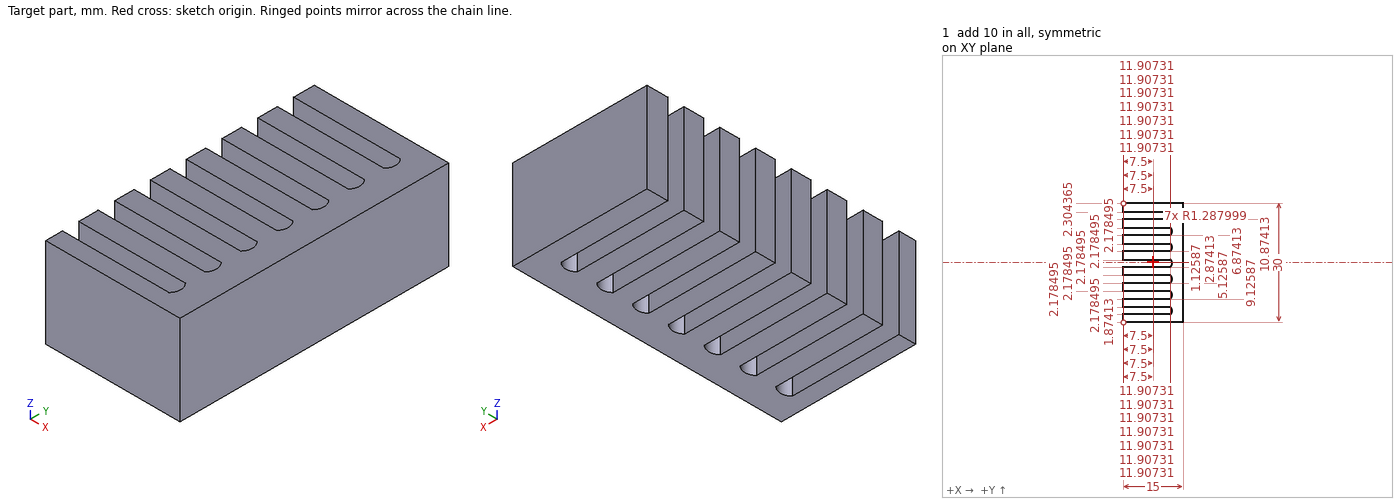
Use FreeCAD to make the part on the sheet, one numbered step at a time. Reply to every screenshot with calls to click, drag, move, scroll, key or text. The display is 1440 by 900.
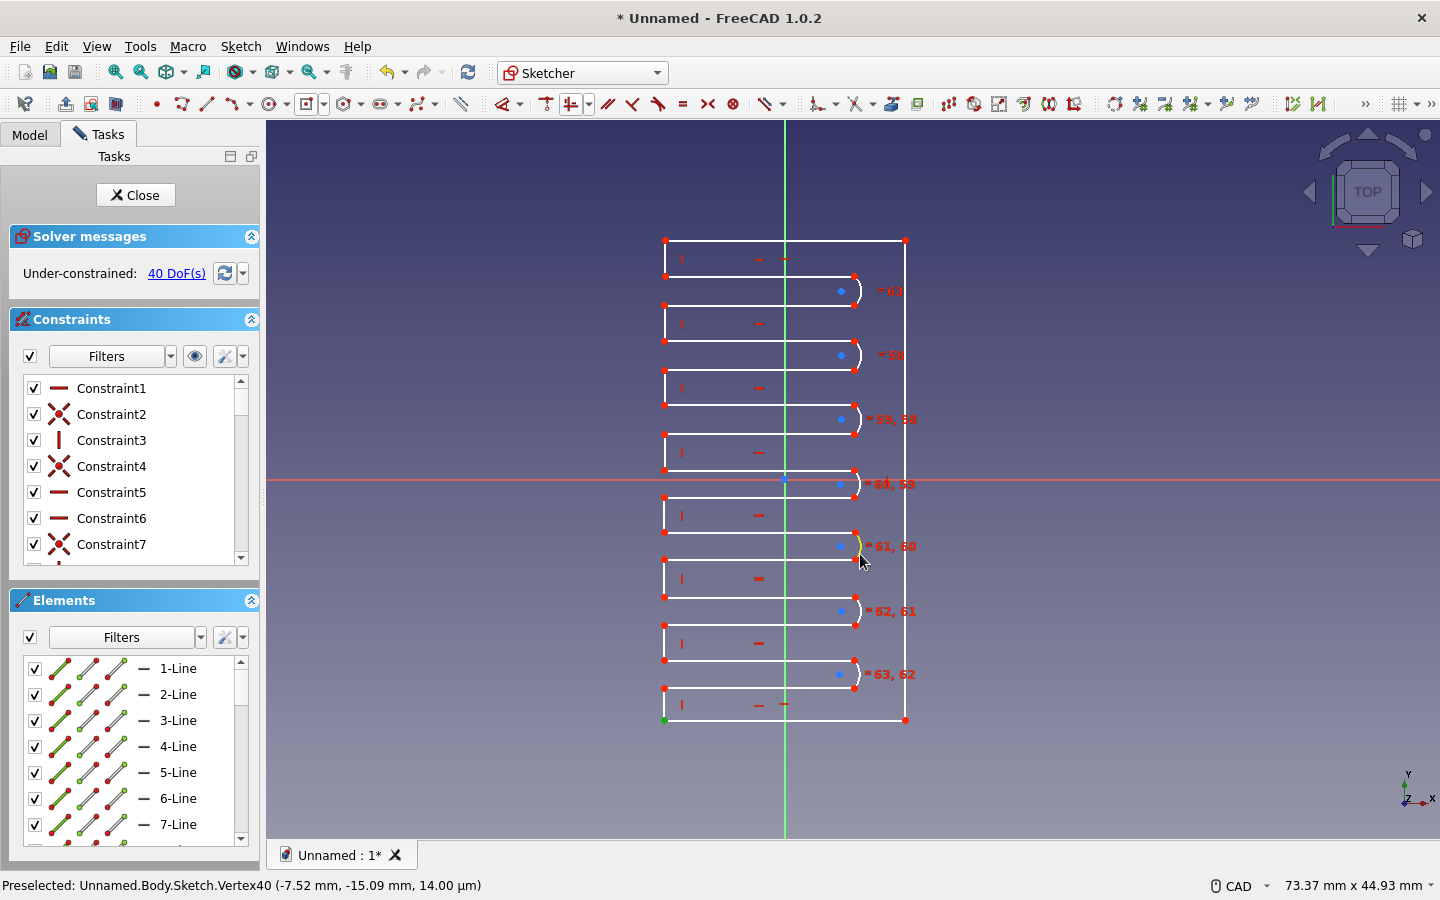
click(665, 241)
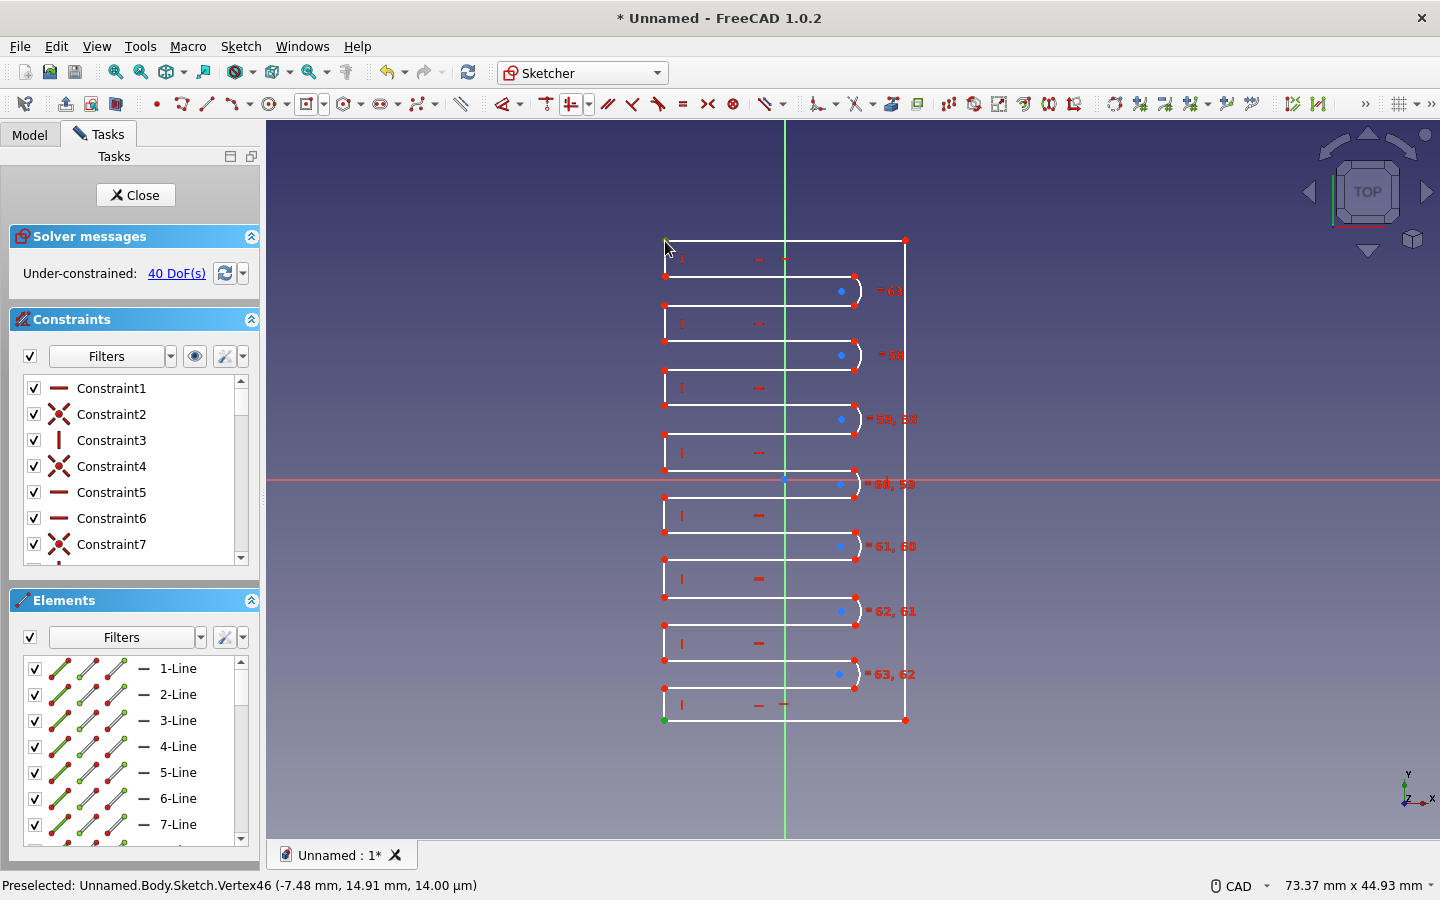
click(364, 480)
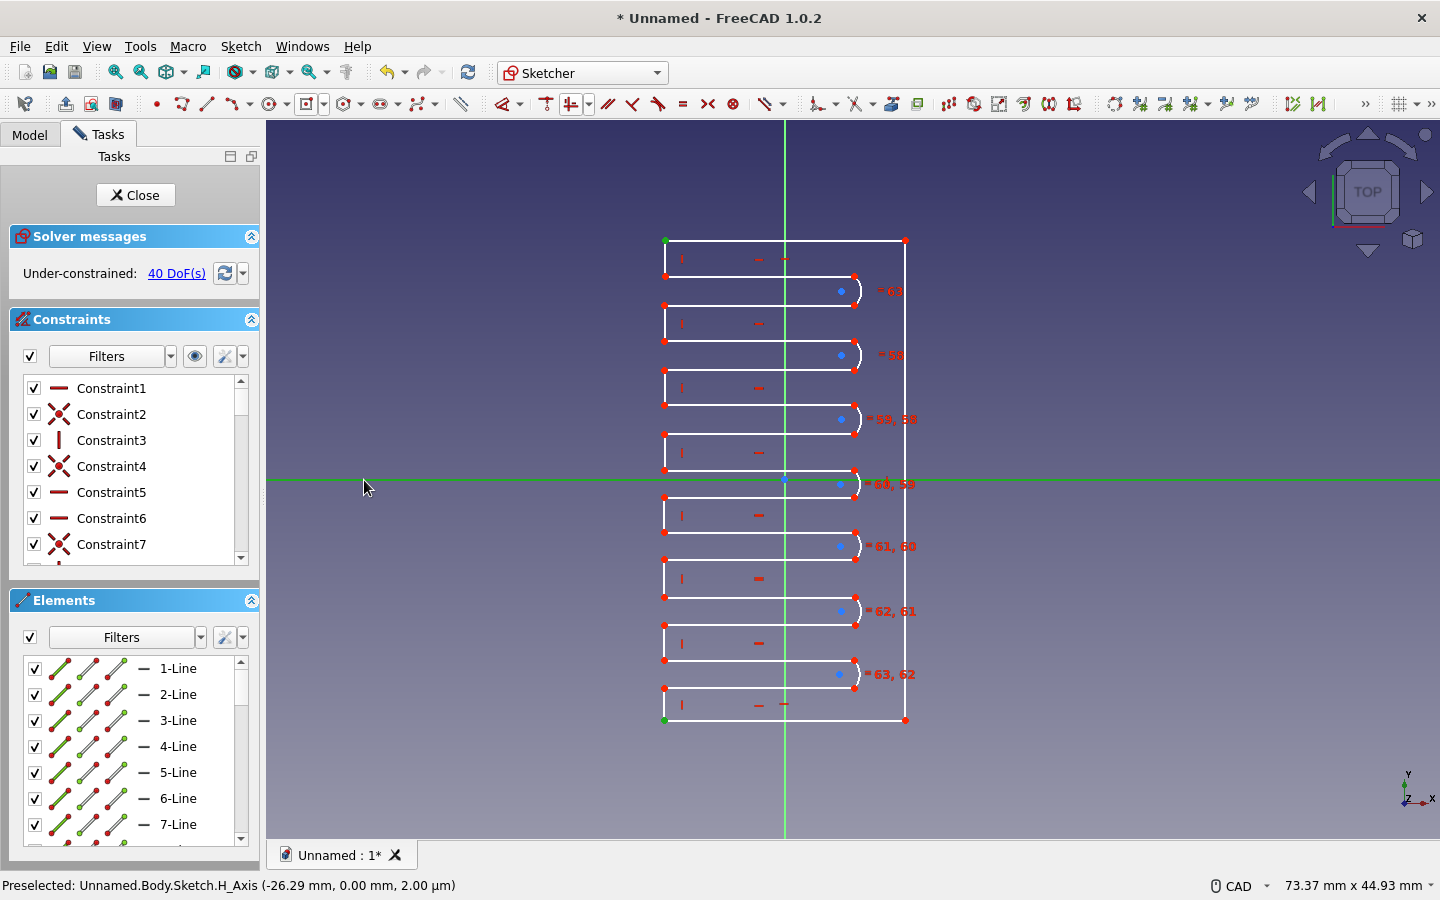
click(708, 104)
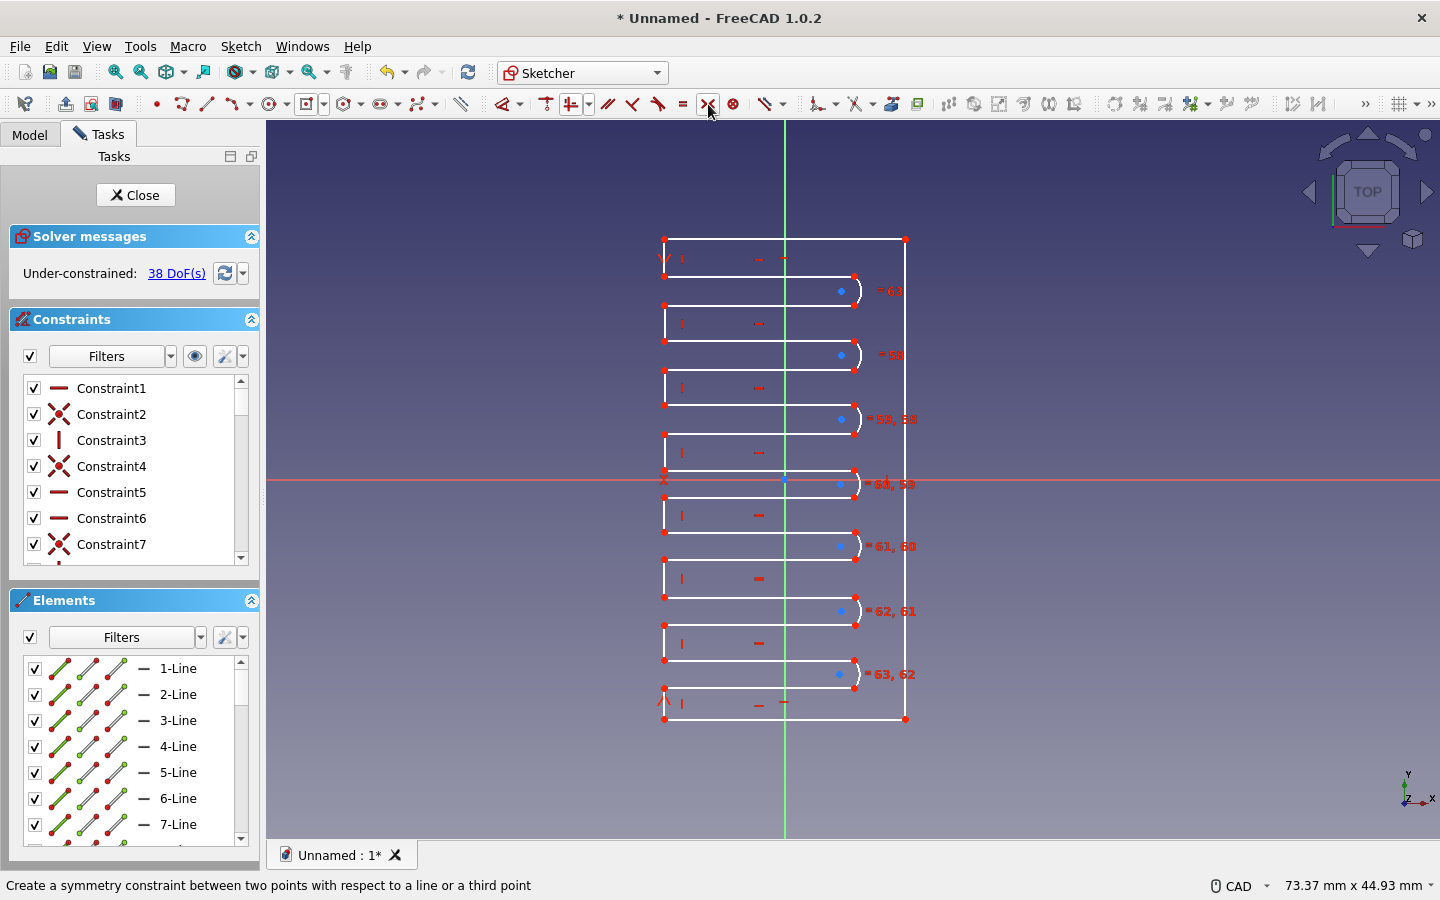
click(502, 104)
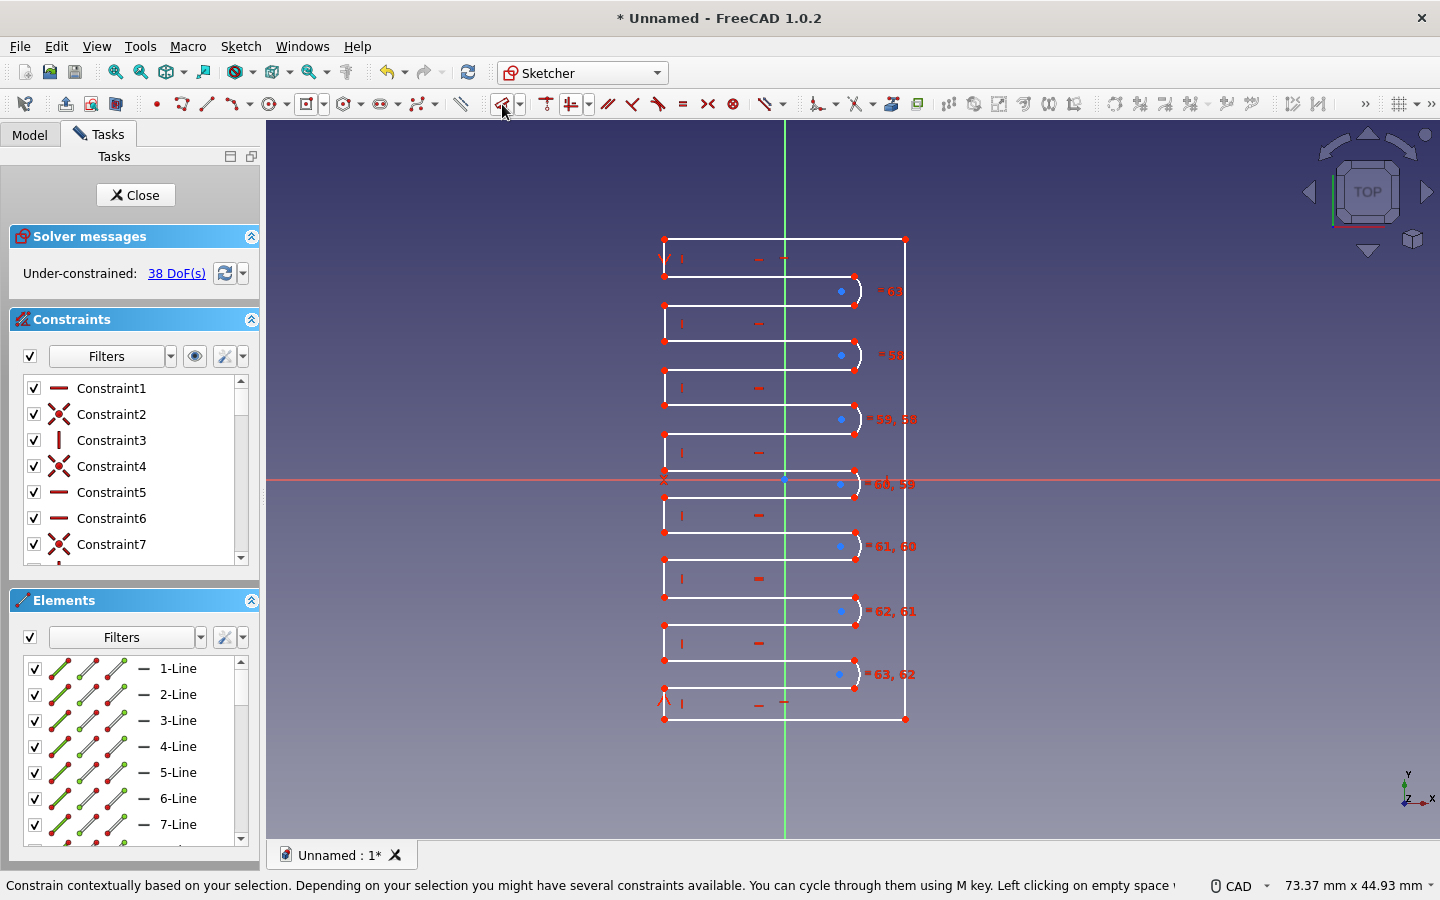
scroll(860, 362, up, 4)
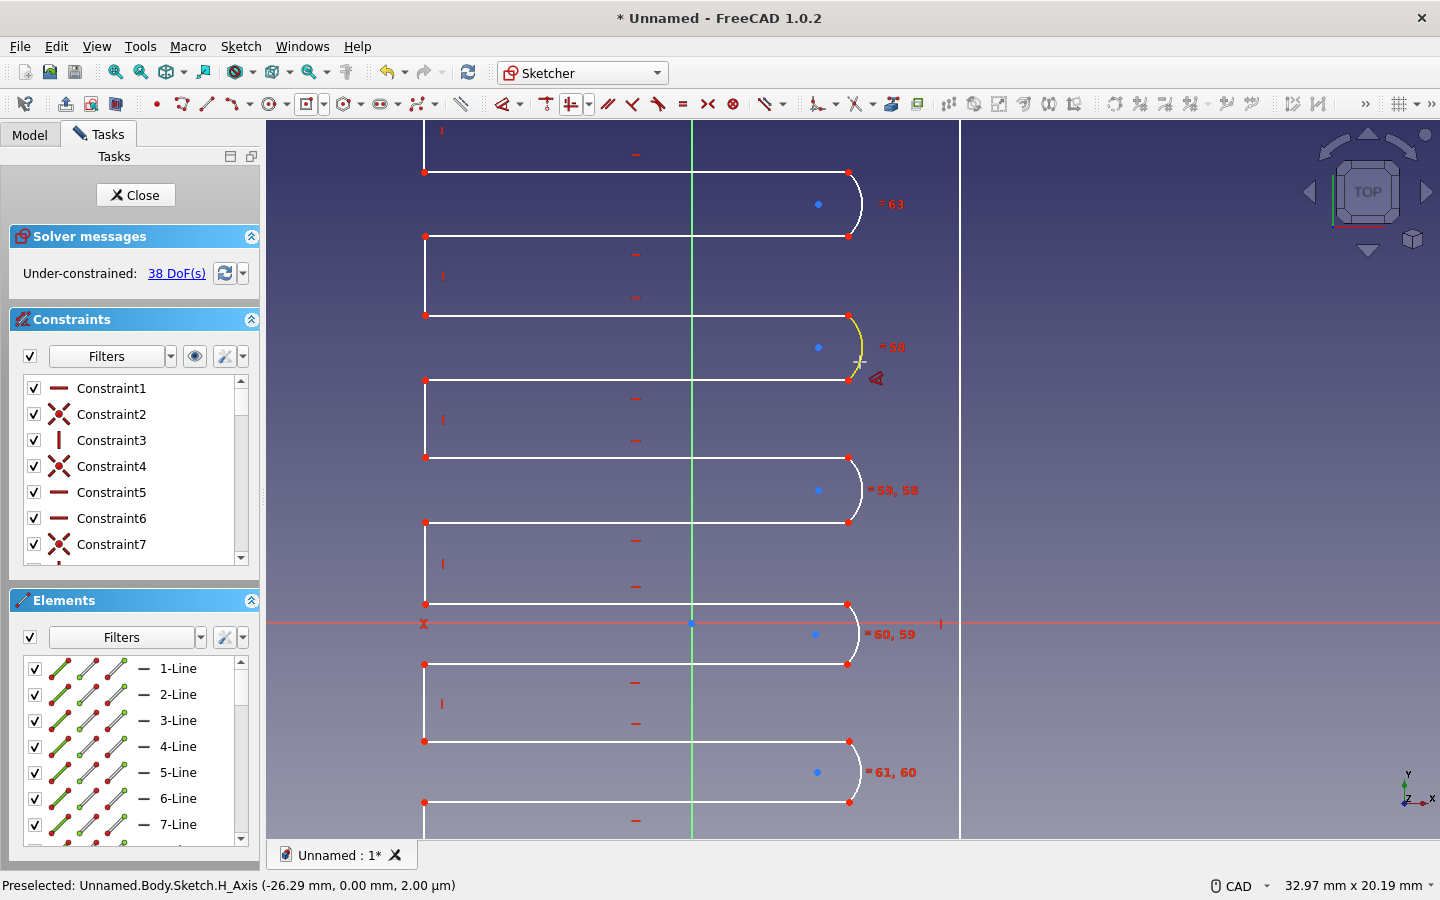
click(860, 362)
click(890, 372)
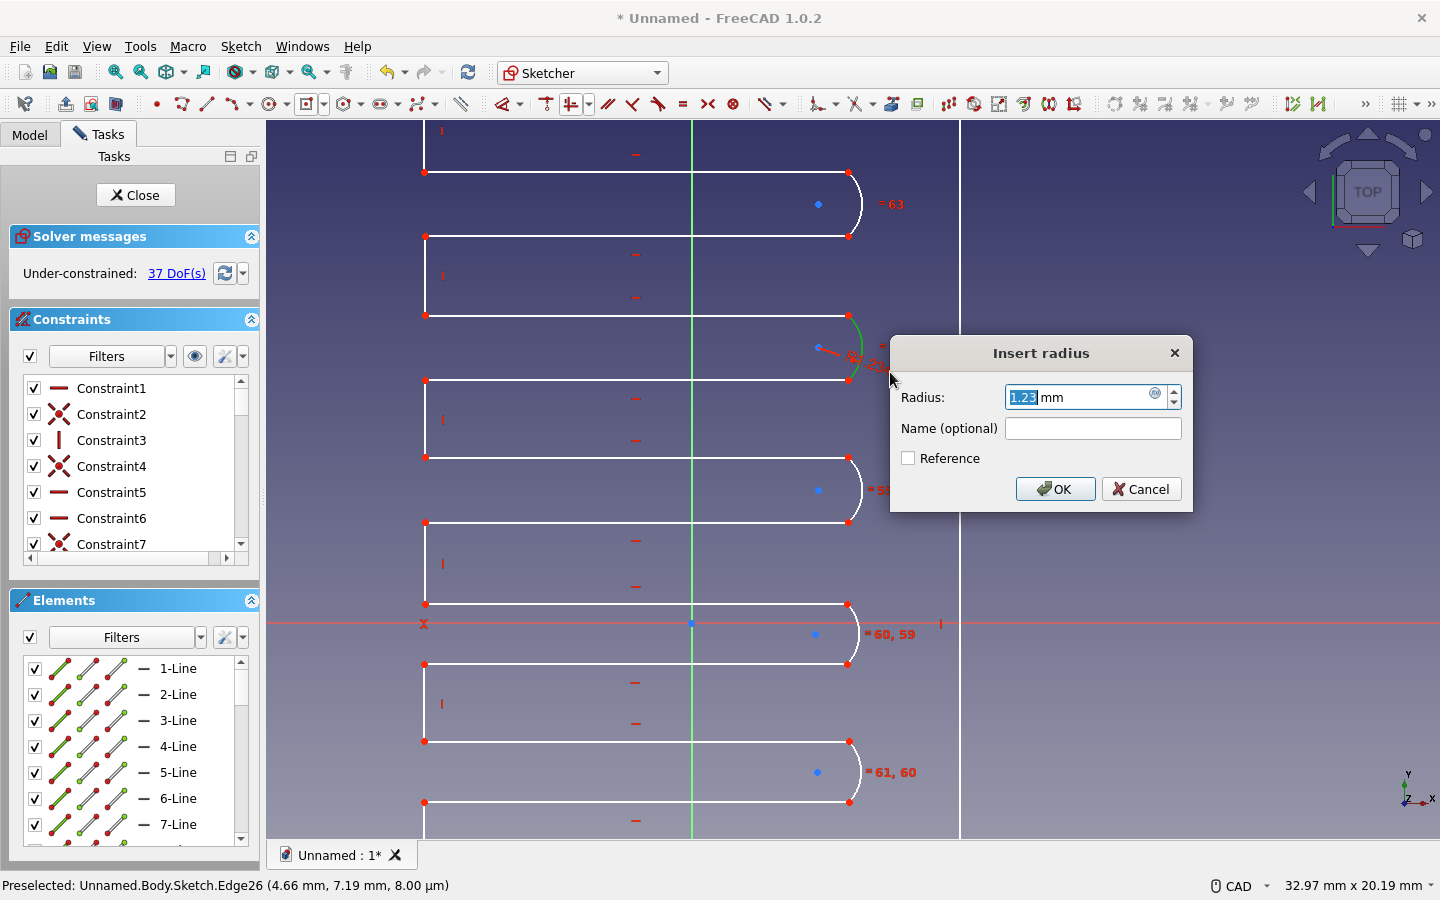
text(1.287999)
key(Return)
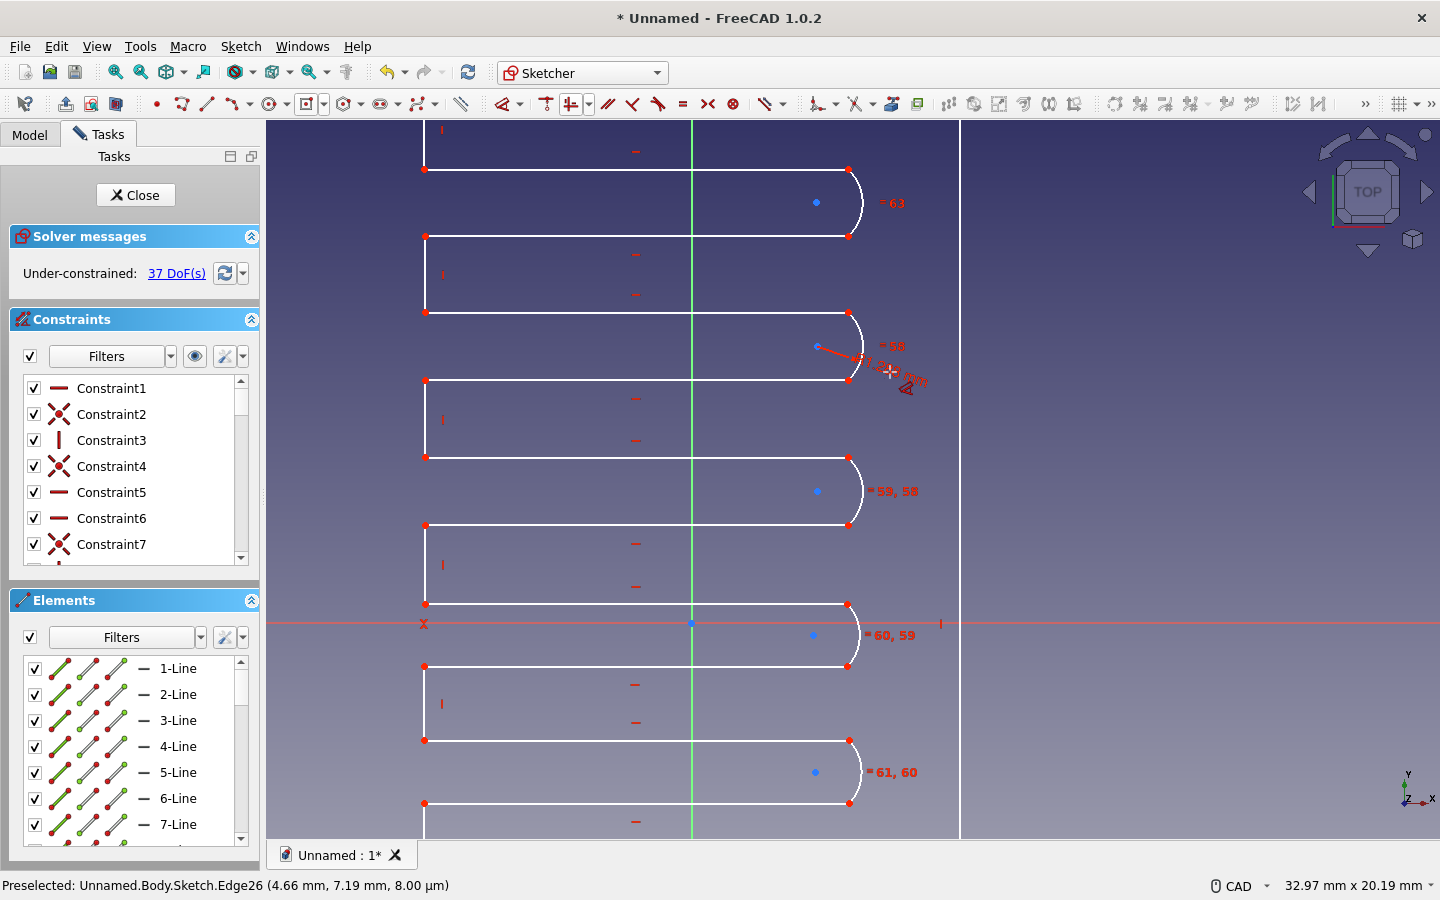
scroll(860, 362, down, 4)